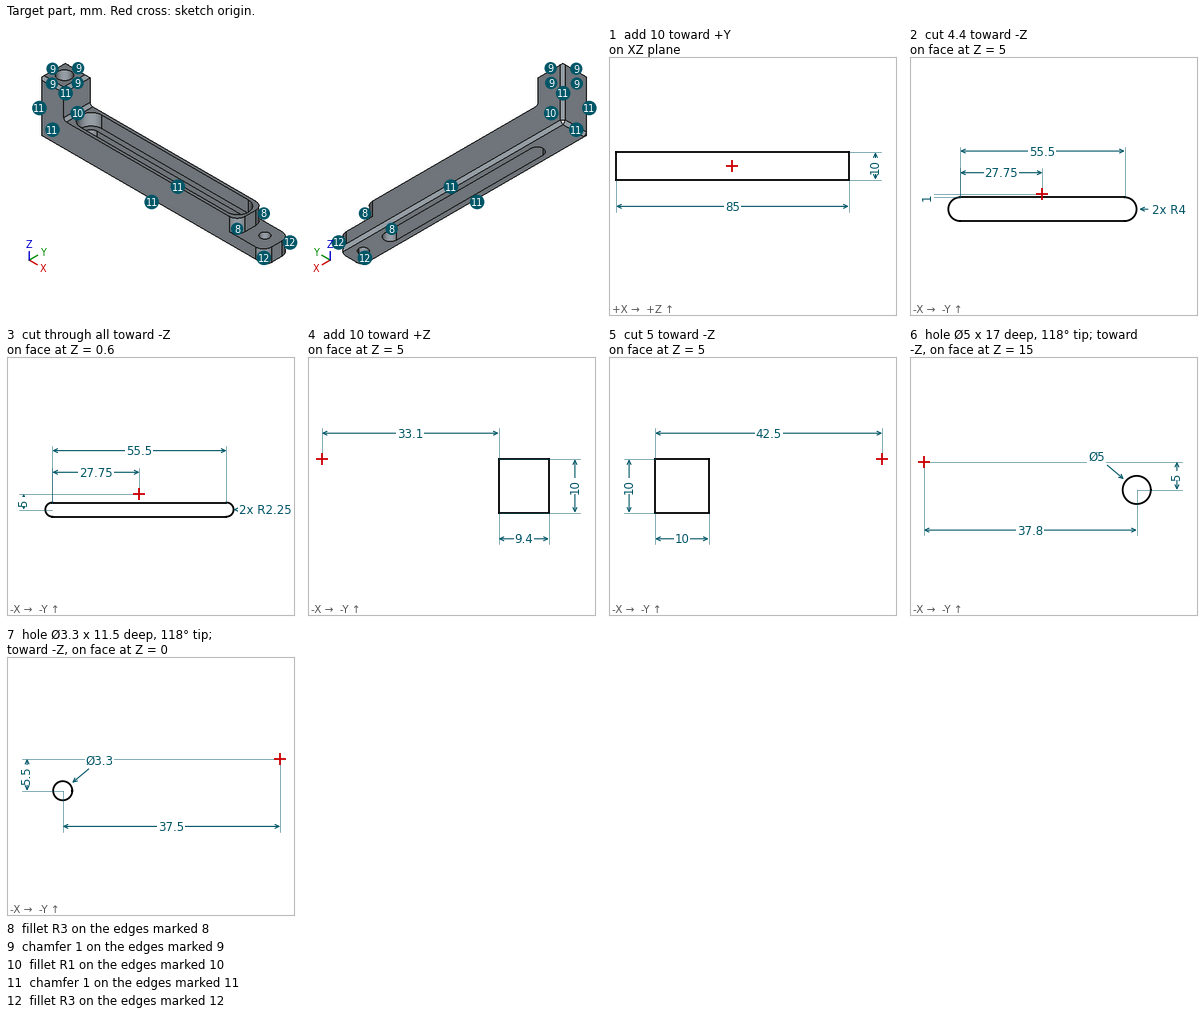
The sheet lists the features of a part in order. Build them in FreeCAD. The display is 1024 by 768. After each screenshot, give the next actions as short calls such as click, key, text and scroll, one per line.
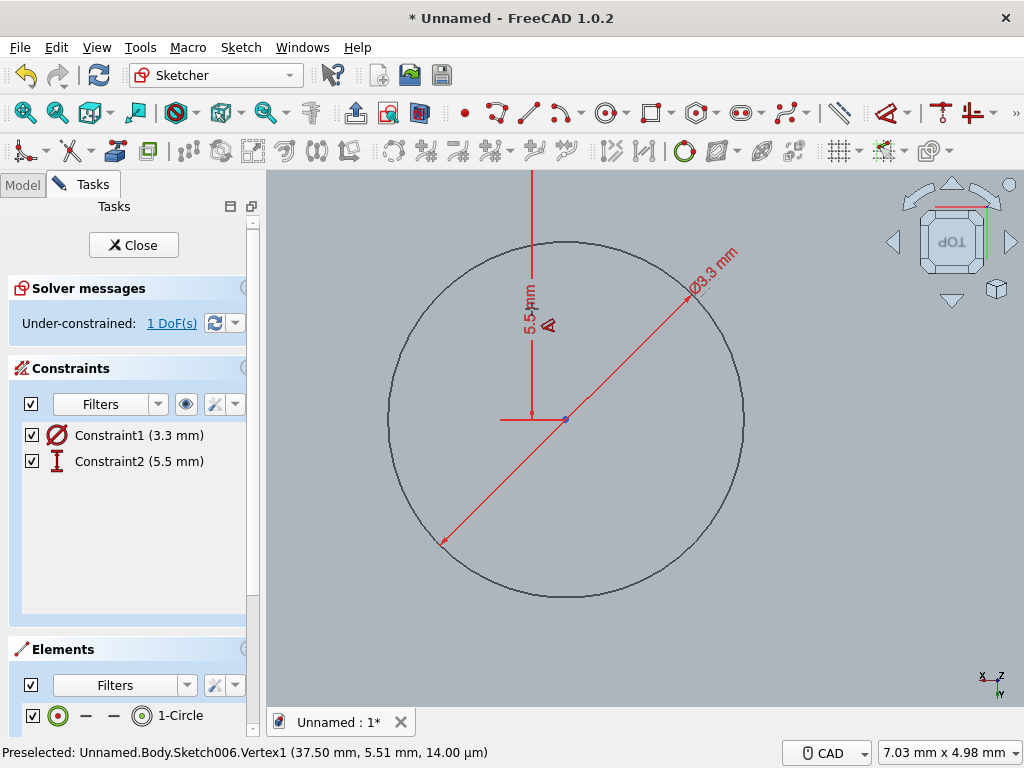
click(566, 420)
click(712, 454)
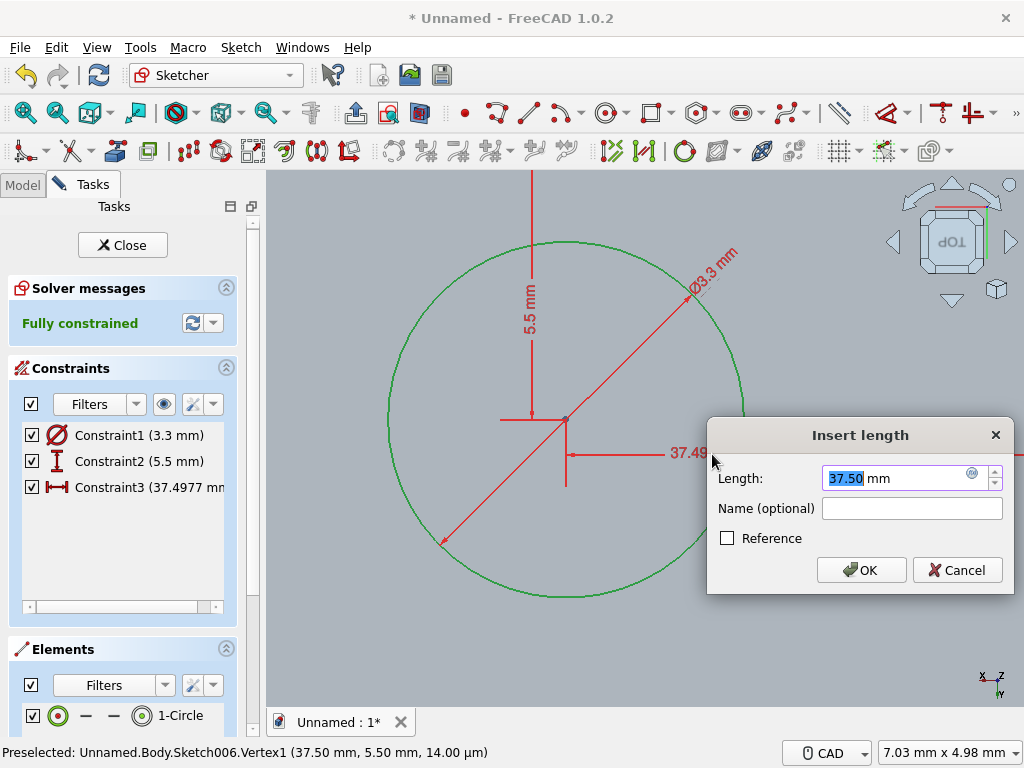
text(37.5)
key(Return)
key(Escape)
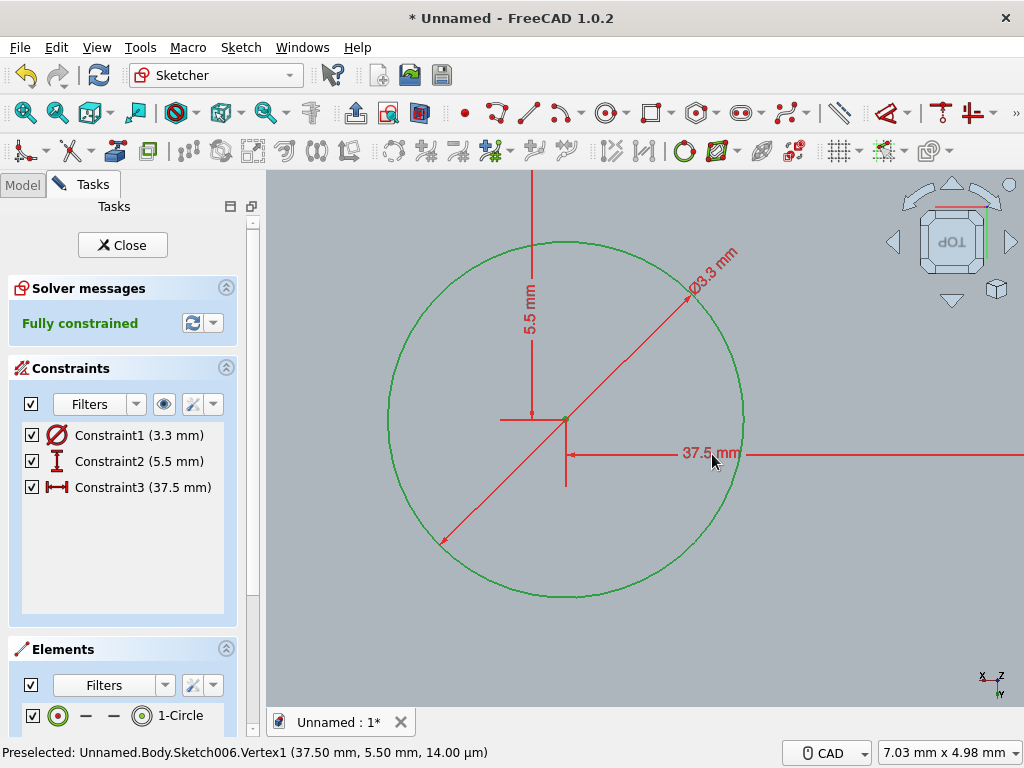
click(123, 245)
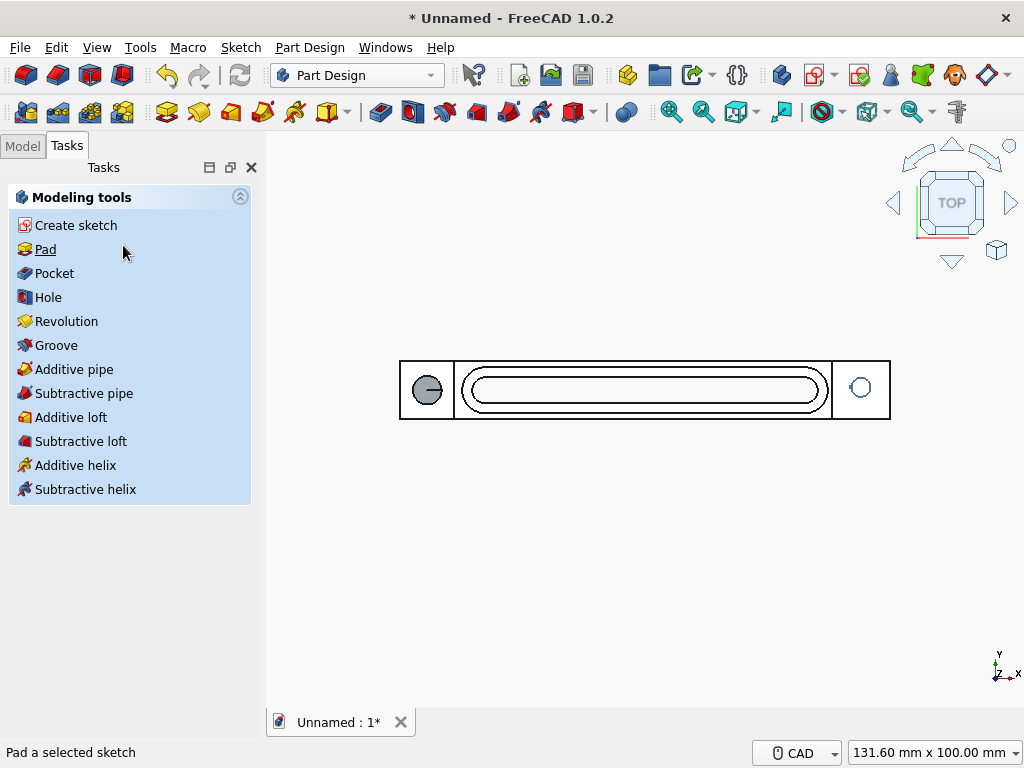
click(414, 112)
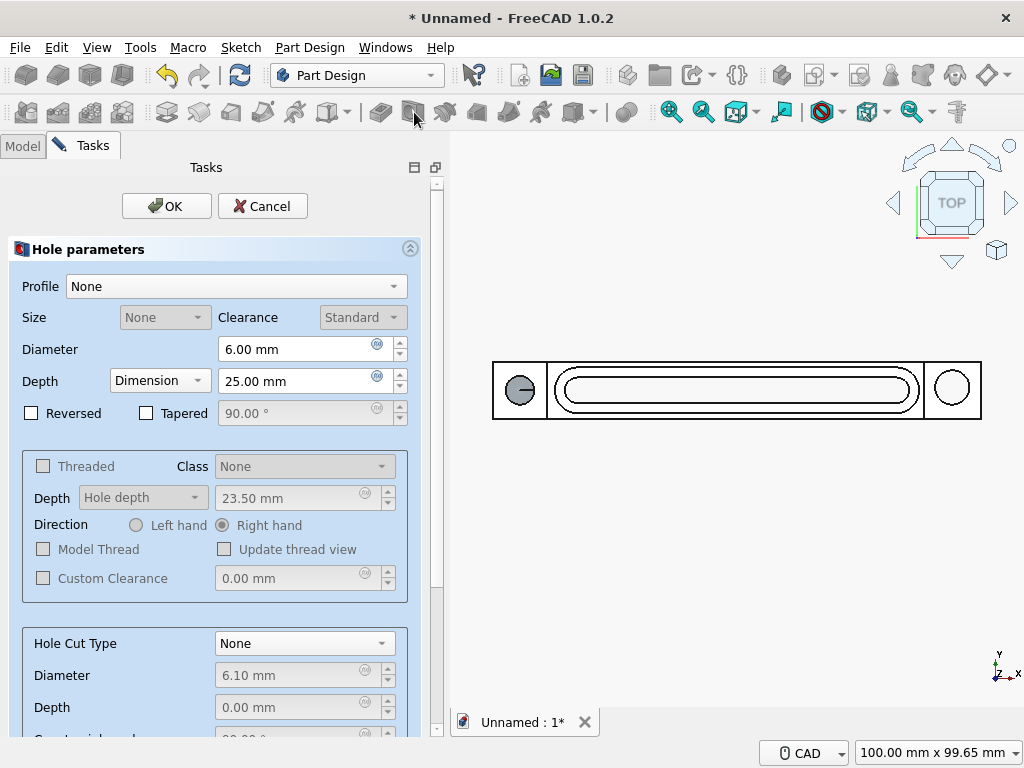
triple_click(305, 349)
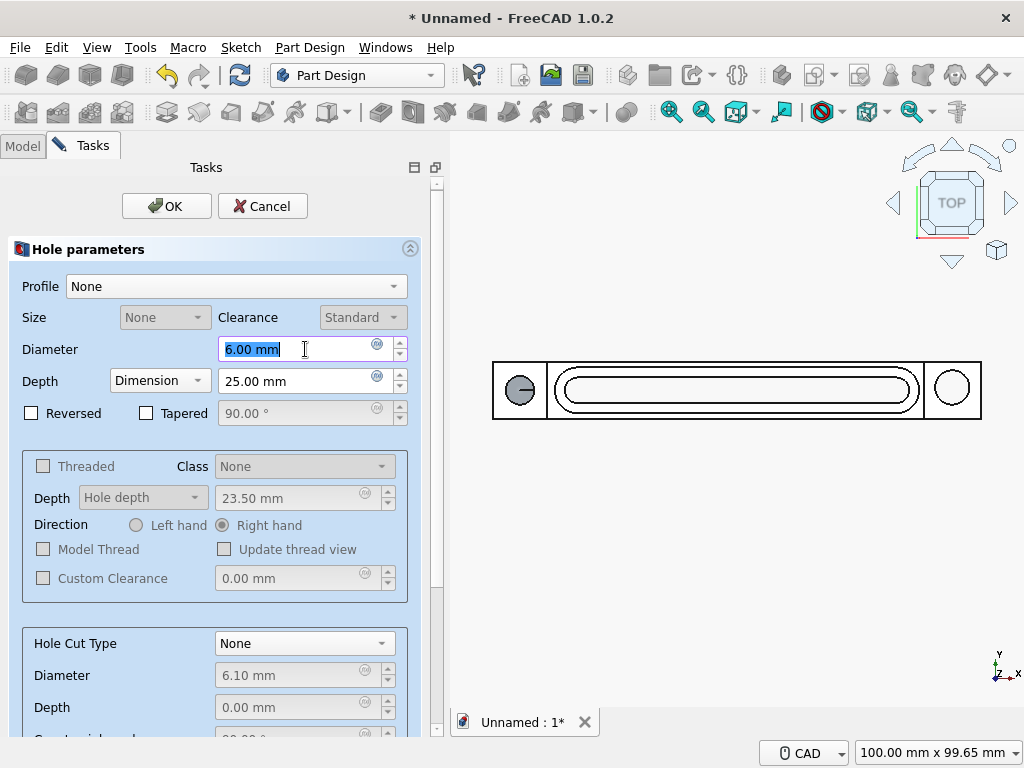
text(3.3)
key(Tab)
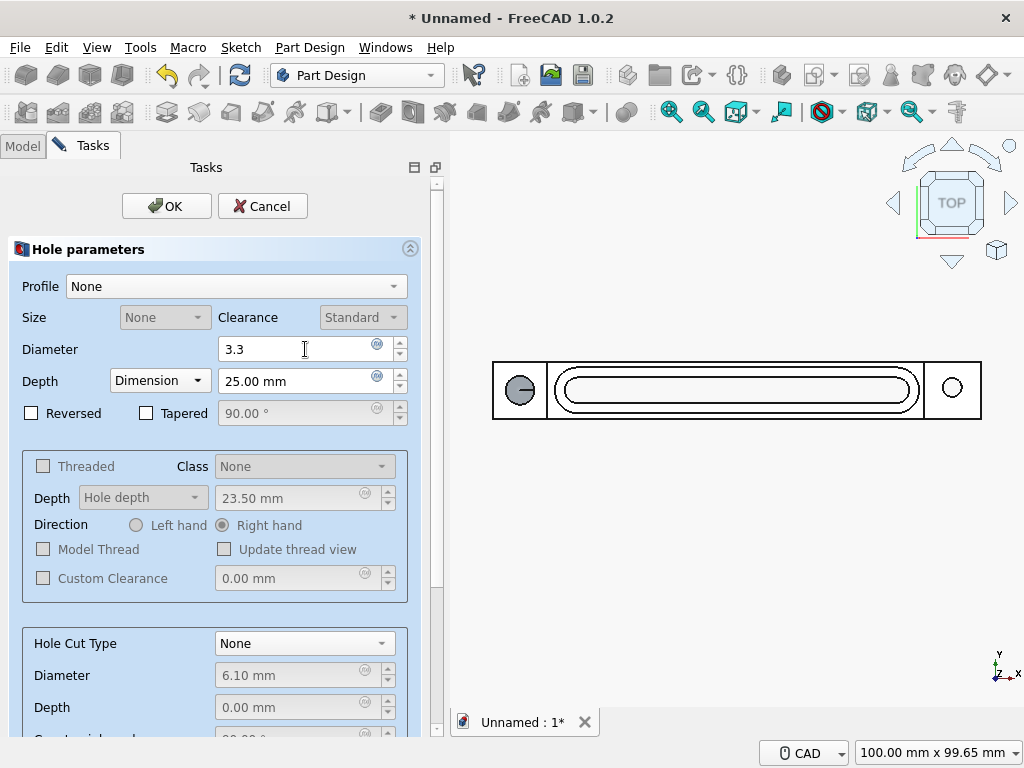
triple_click(305, 381)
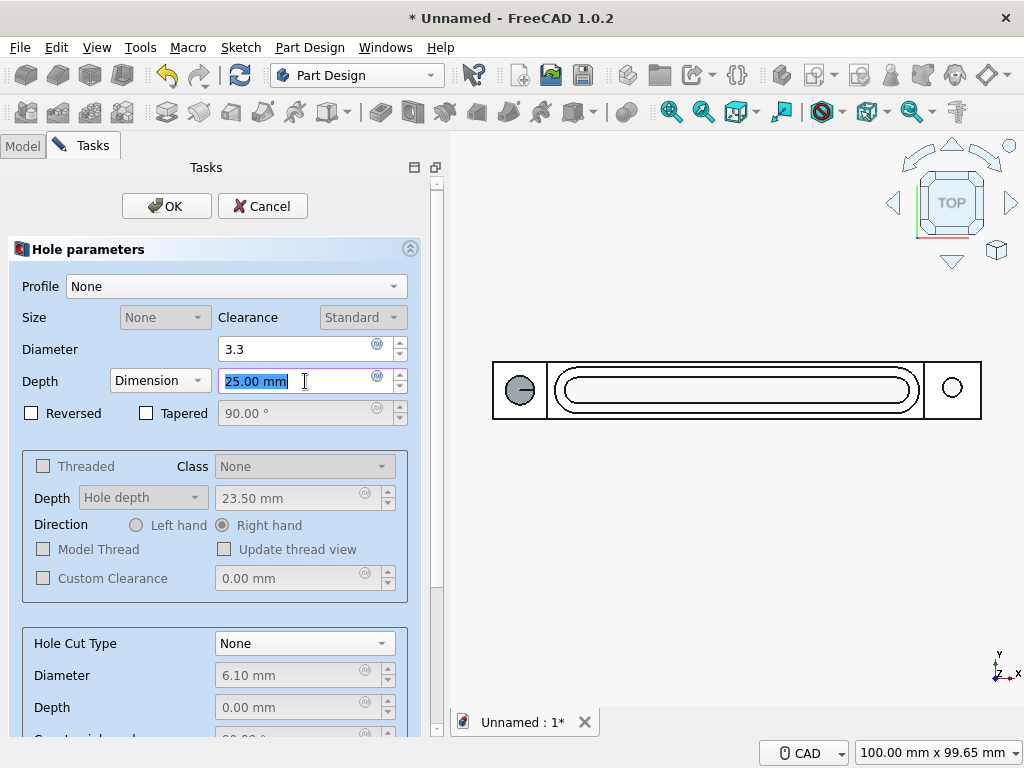
text(11.5)
key(Tab)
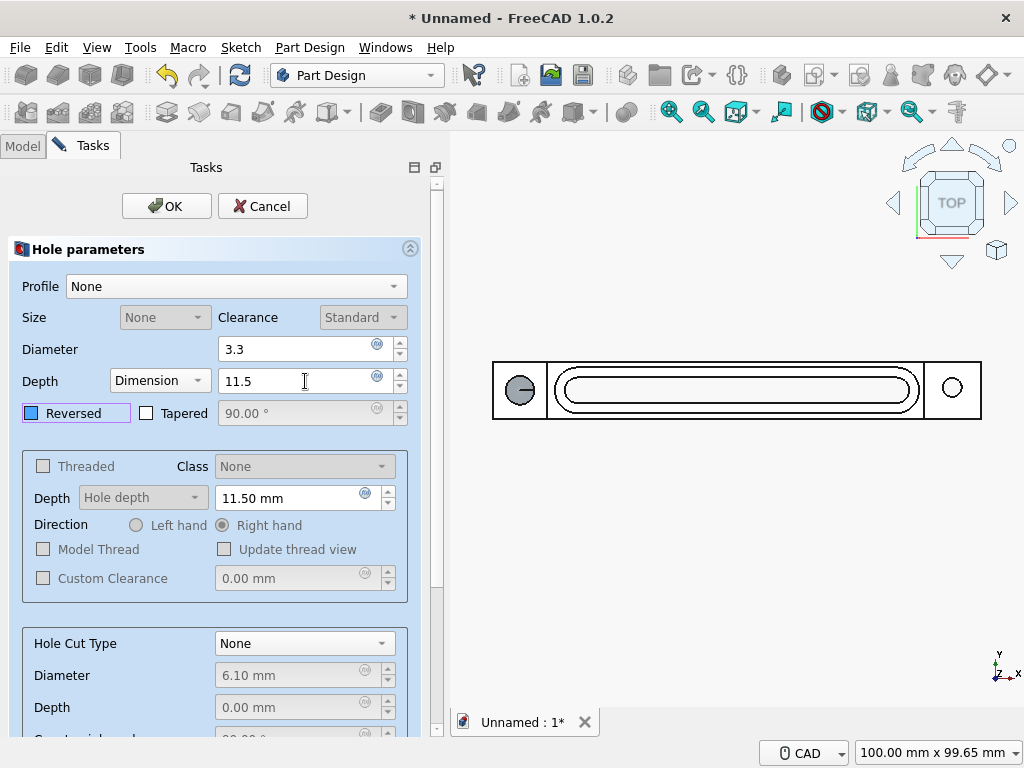
click(167, 206)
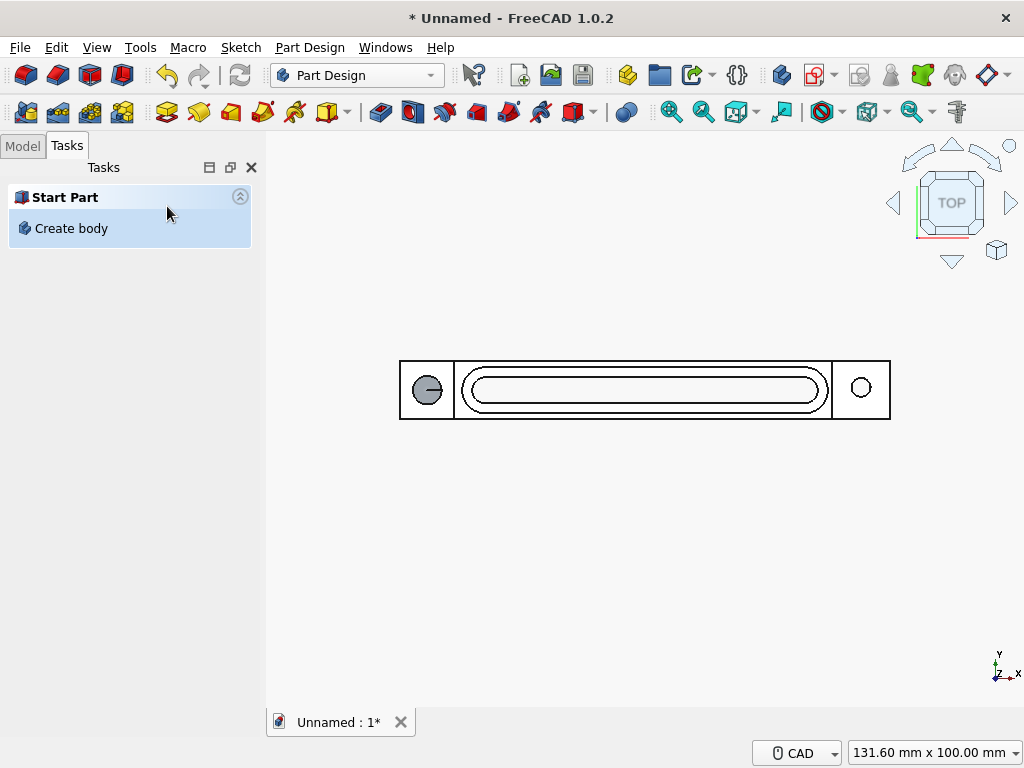
key(0)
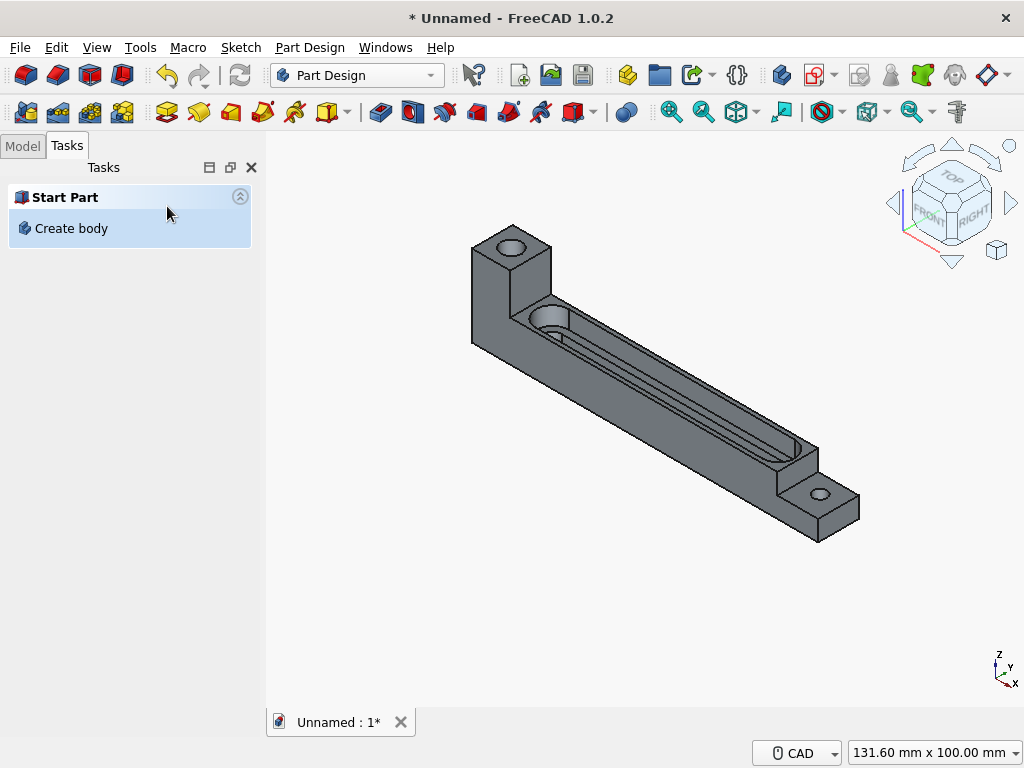
click(777, 483)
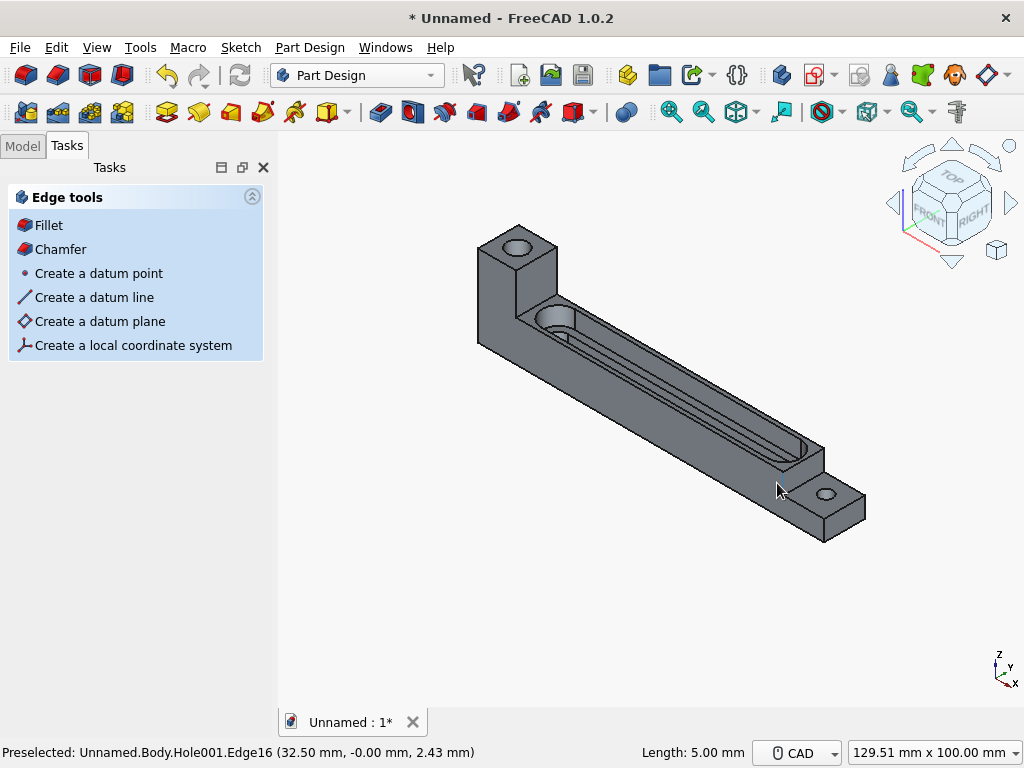
key(2)